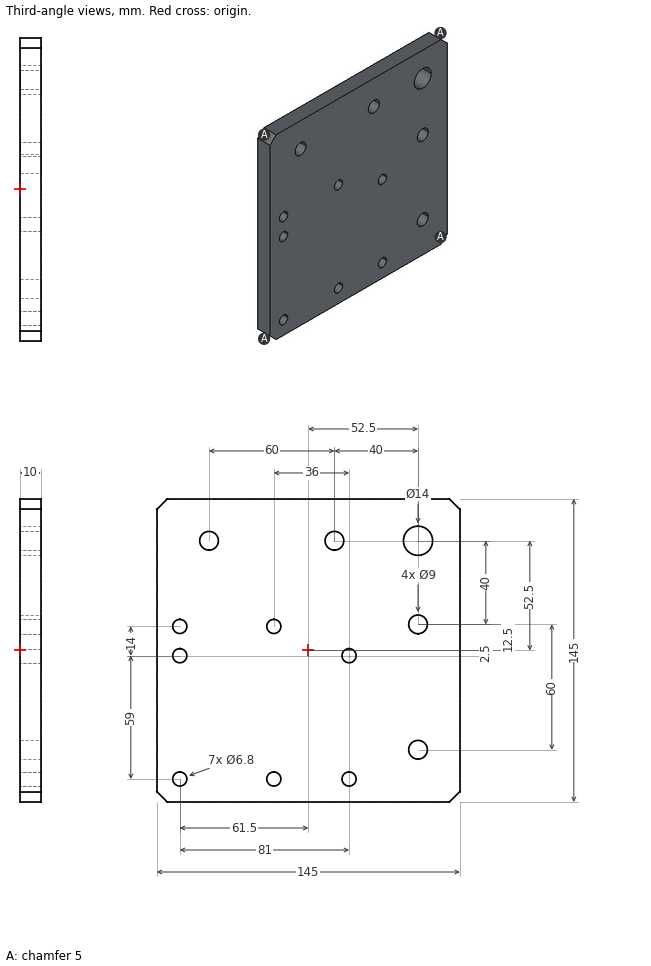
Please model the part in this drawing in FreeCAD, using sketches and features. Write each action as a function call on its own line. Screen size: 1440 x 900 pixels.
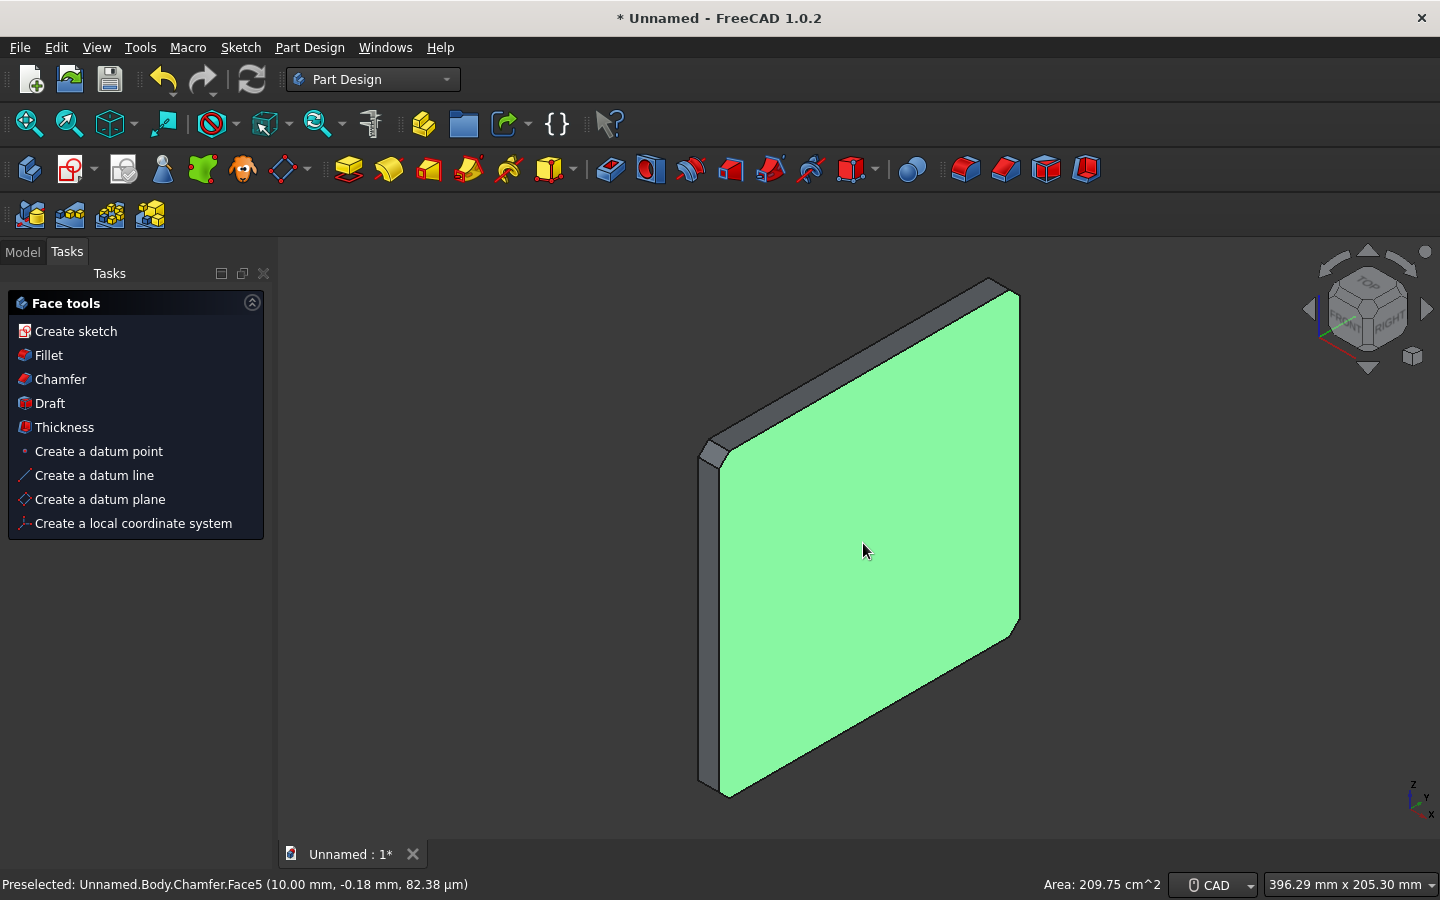
click(70, 170)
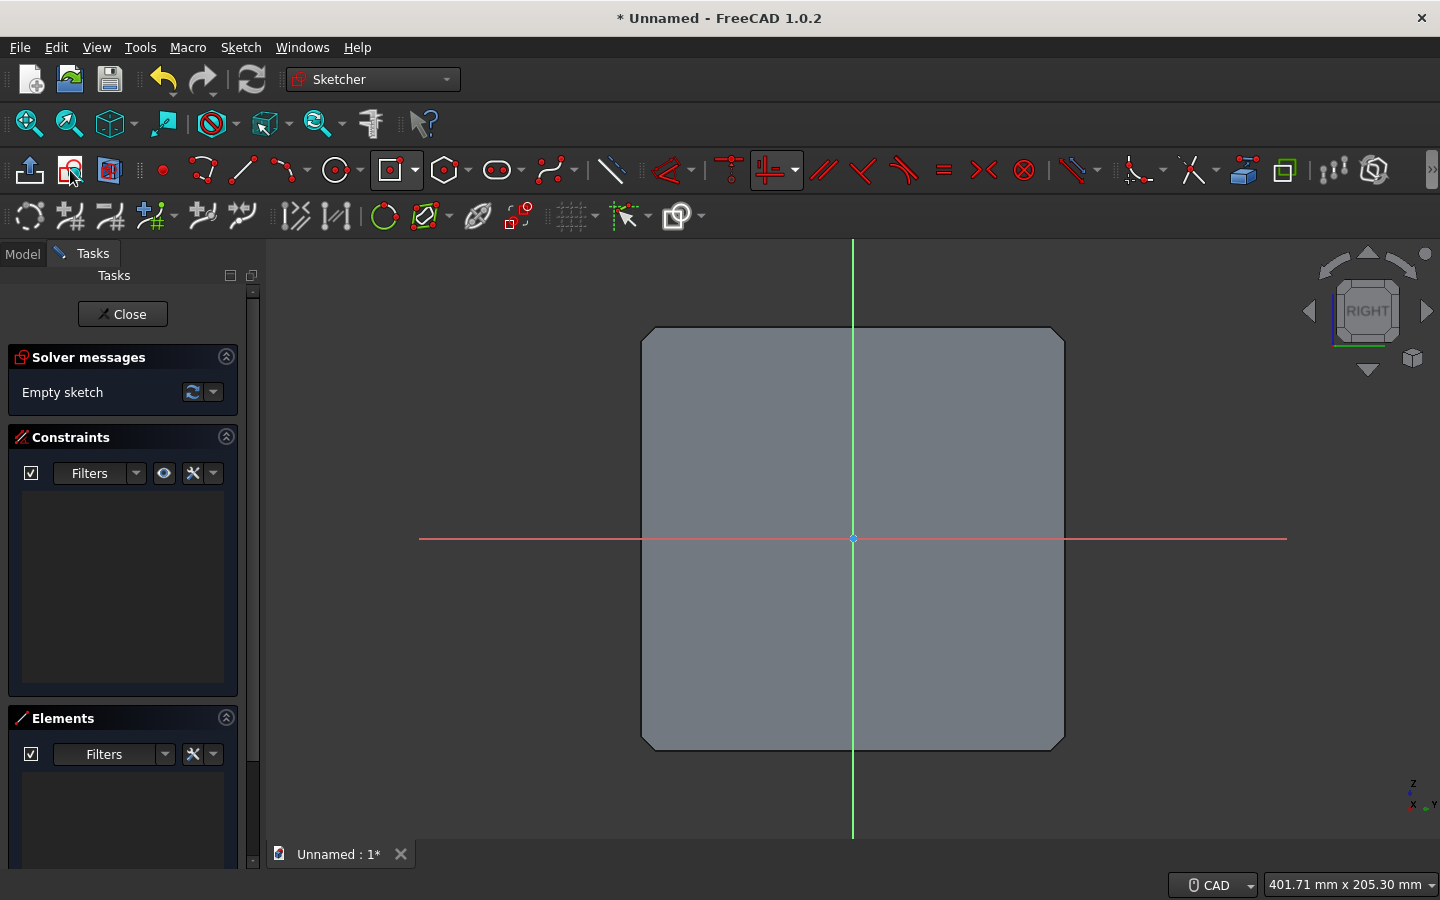
scroll(806, 761, up, 2)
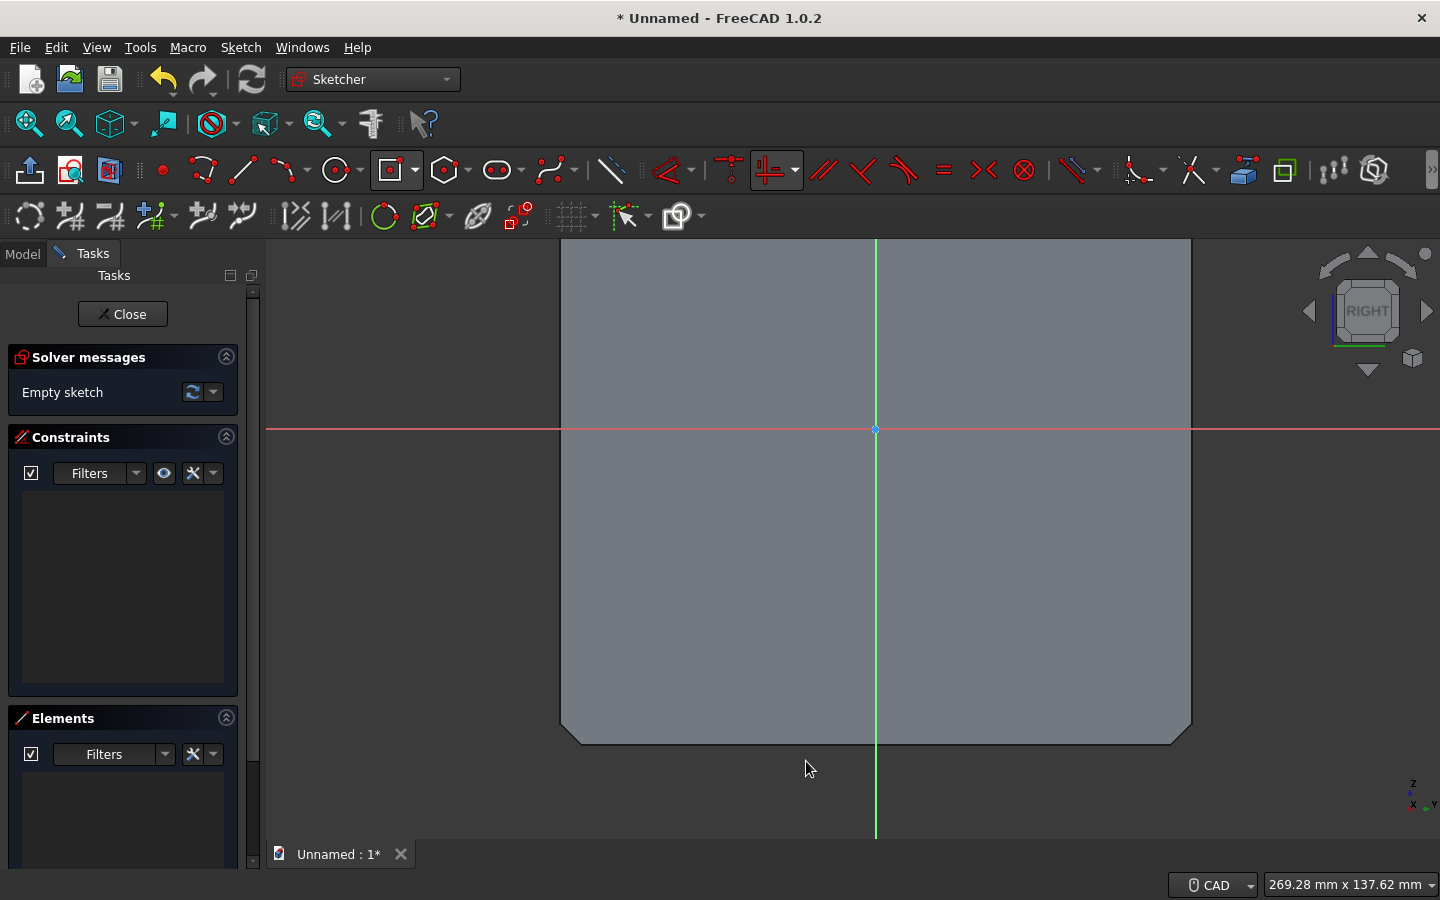
key(g)
key(c)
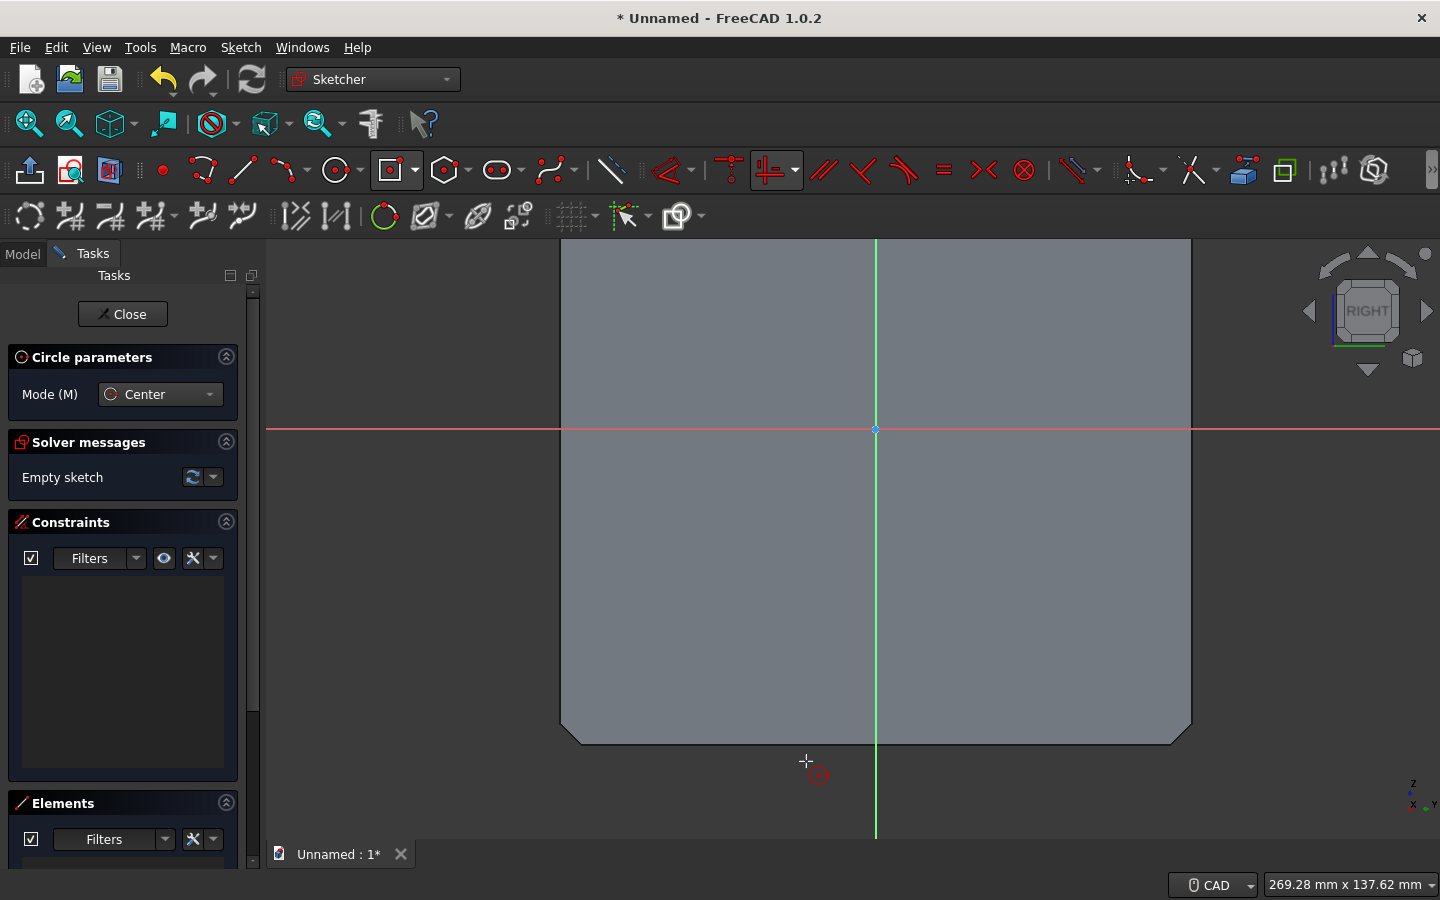
scroll(608, 698, up, 3)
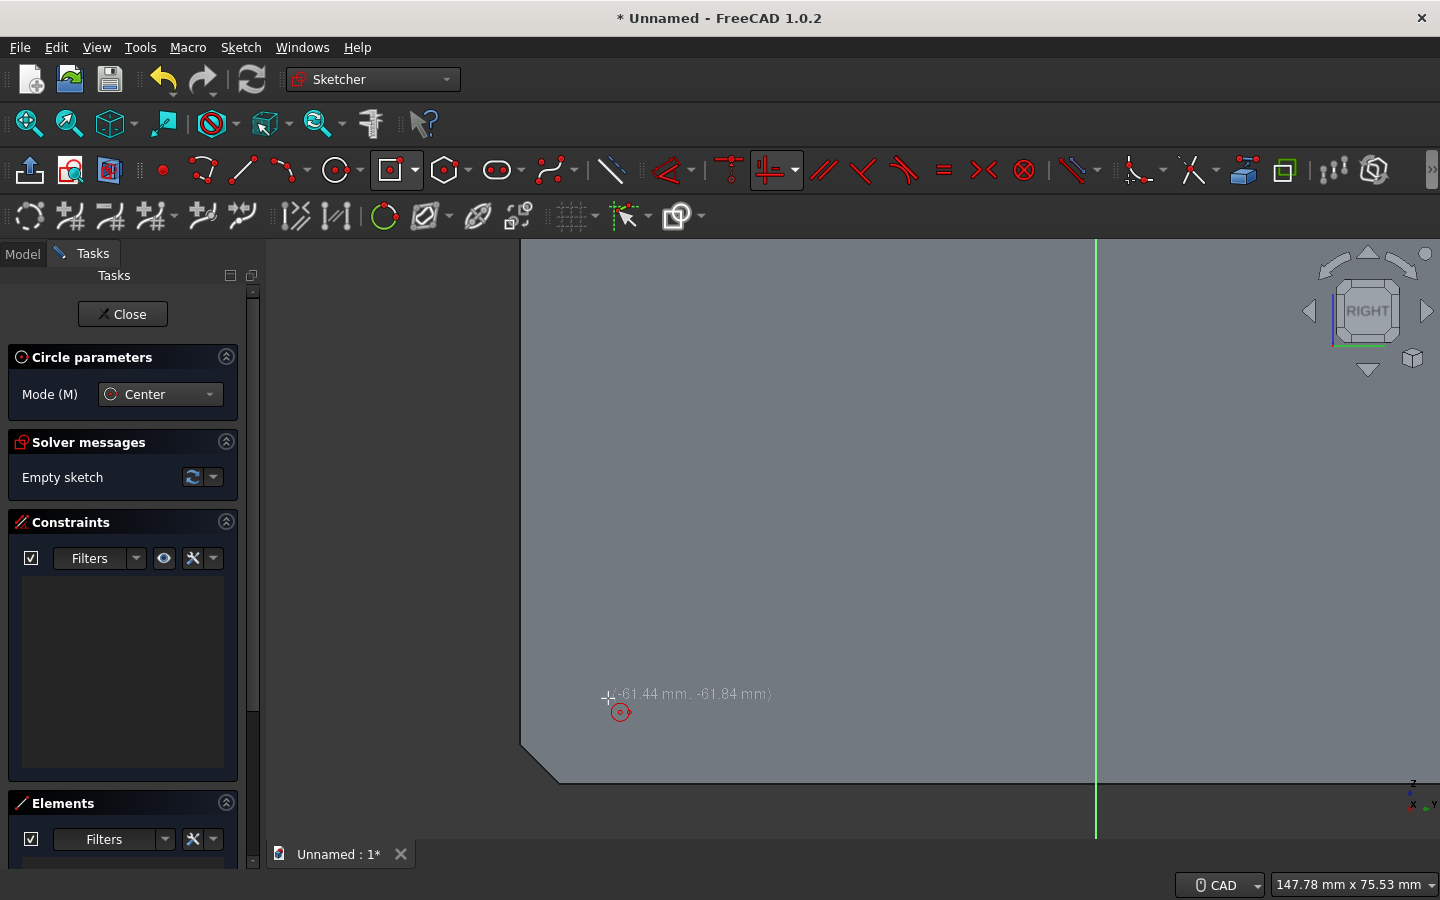
click(607, 696)
click(626, 677)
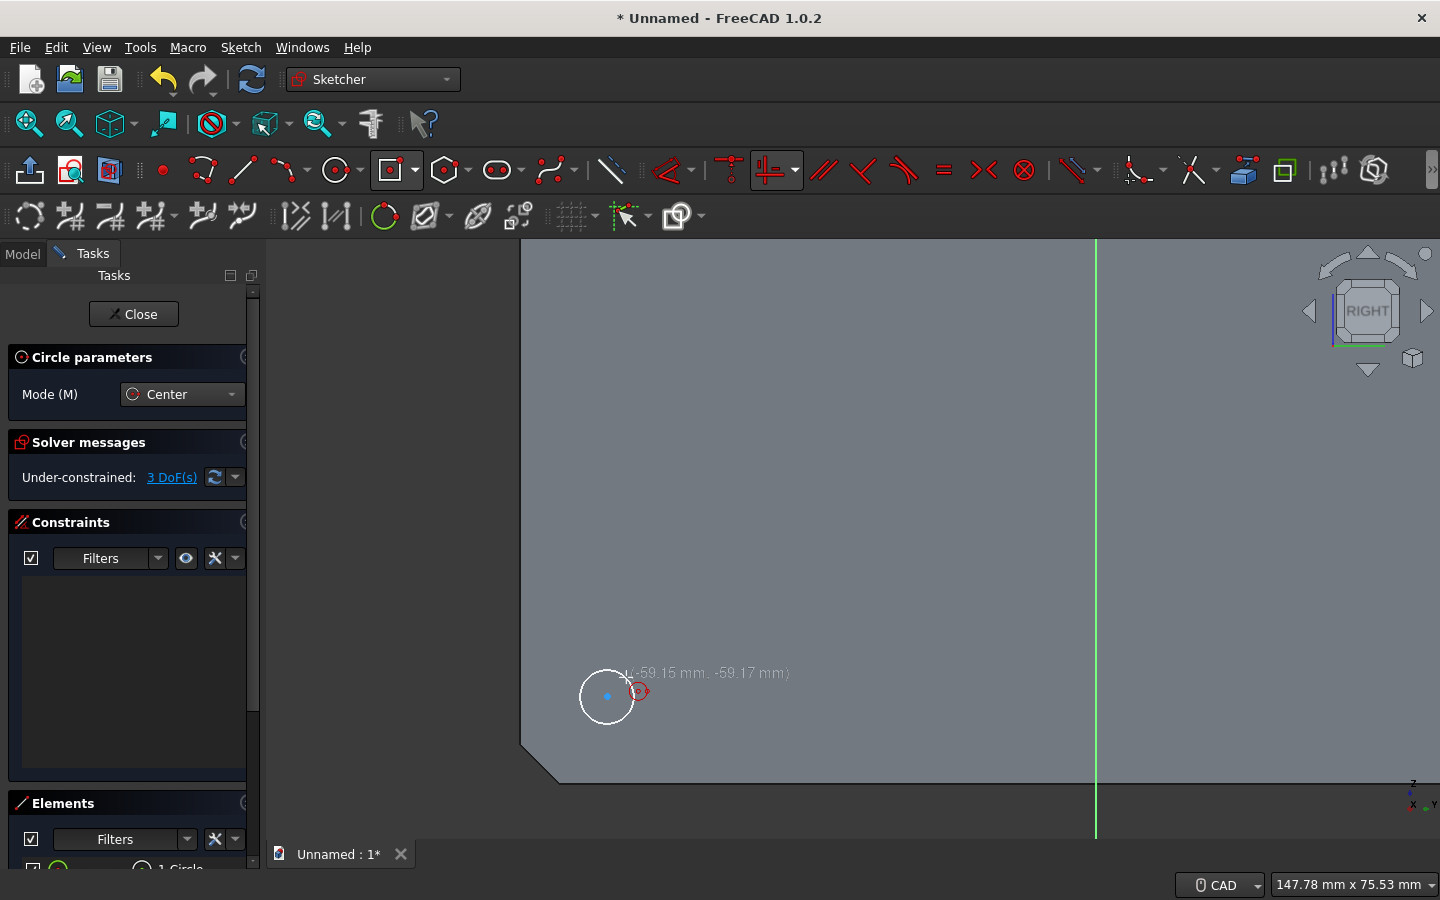
scroll(609, 700, down, 3)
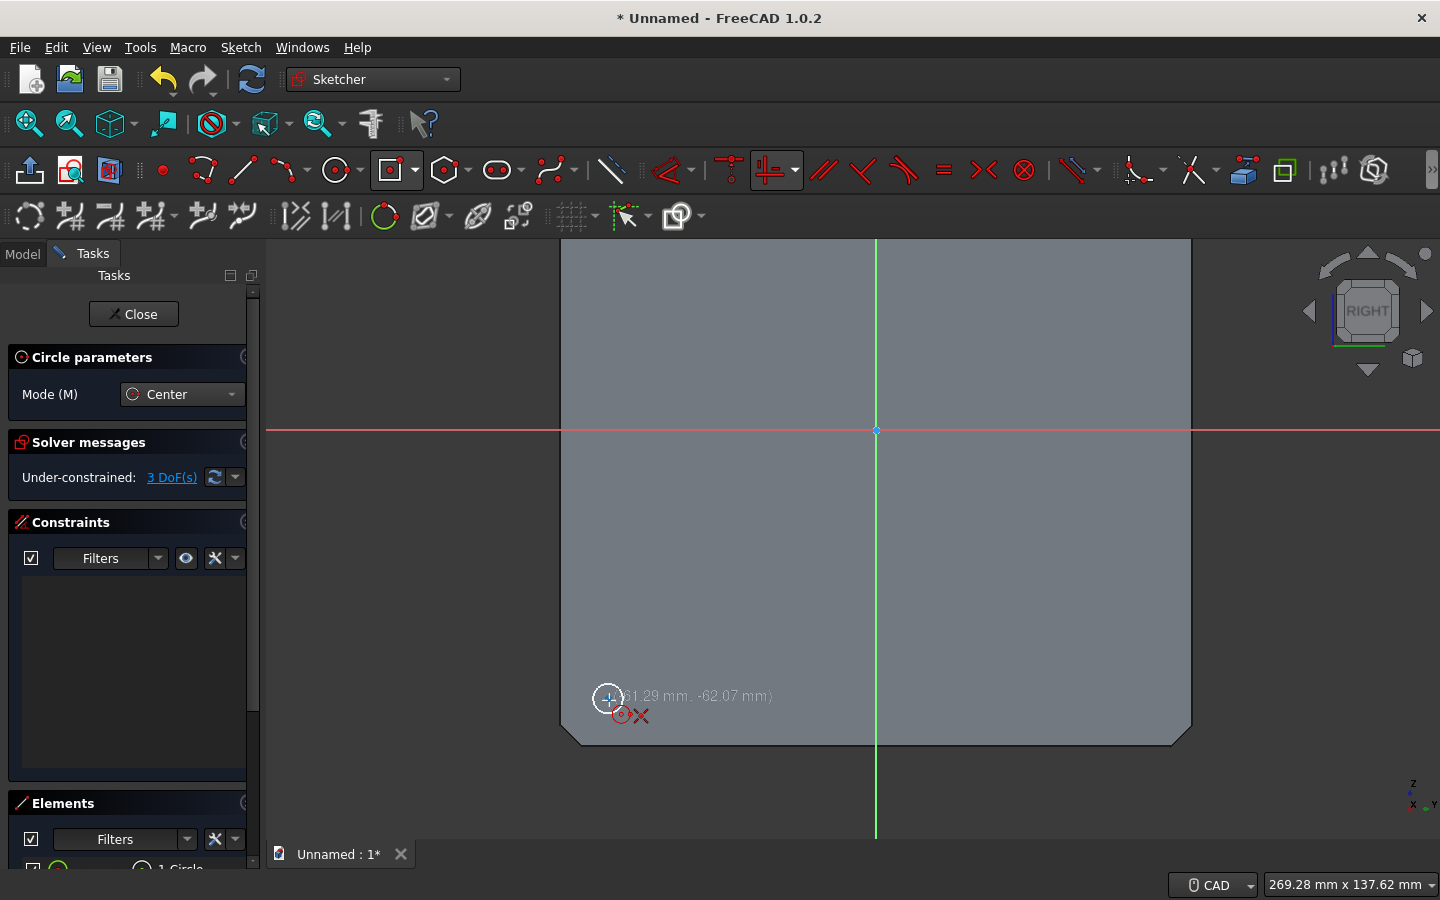
scroll(961, 441, up, 3)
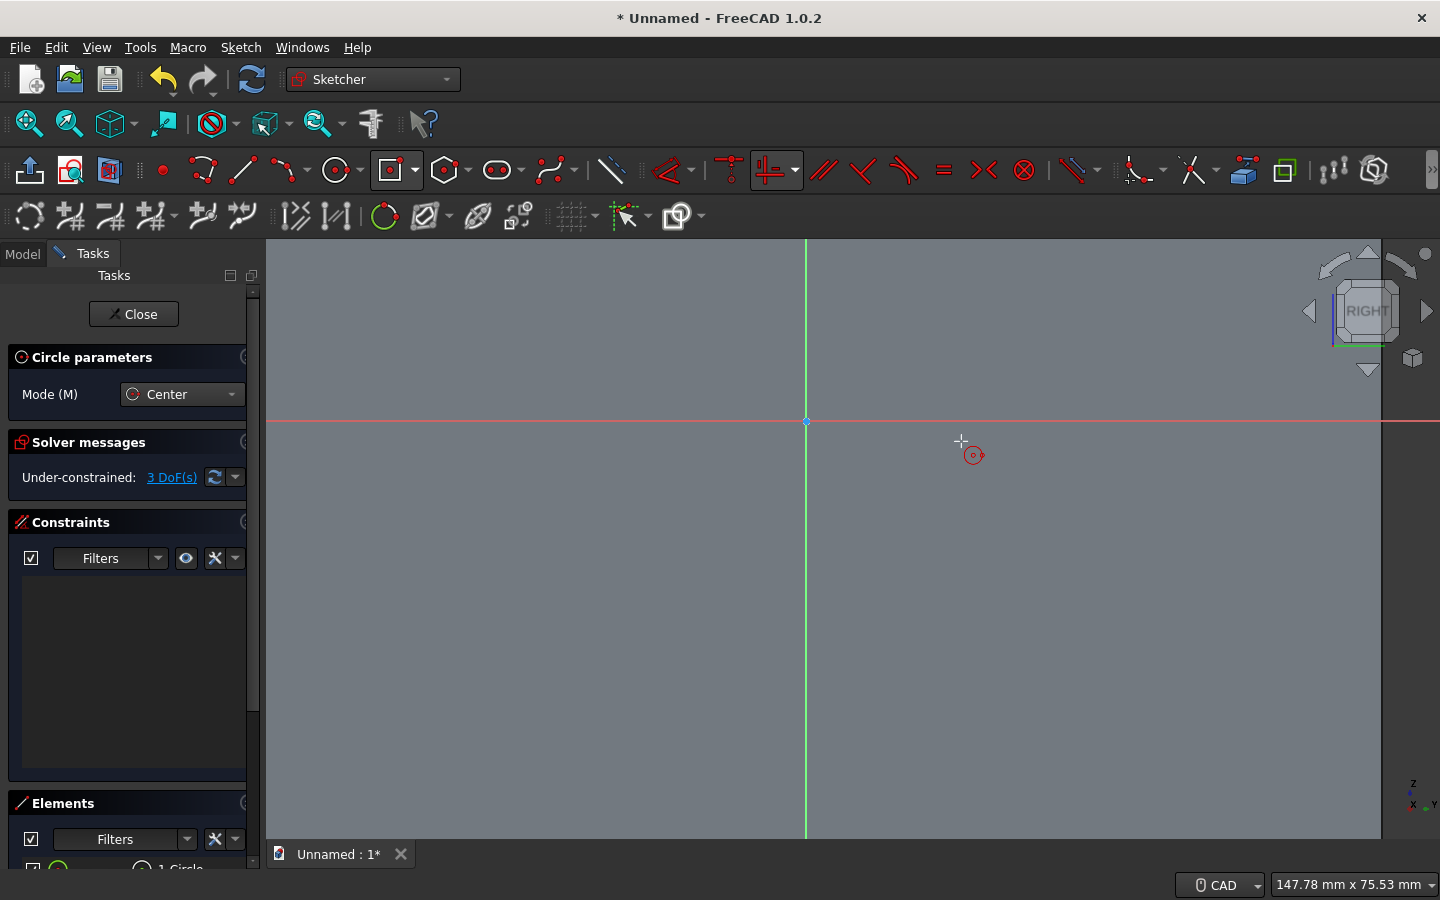
click(961, 441)
click(980, 460)